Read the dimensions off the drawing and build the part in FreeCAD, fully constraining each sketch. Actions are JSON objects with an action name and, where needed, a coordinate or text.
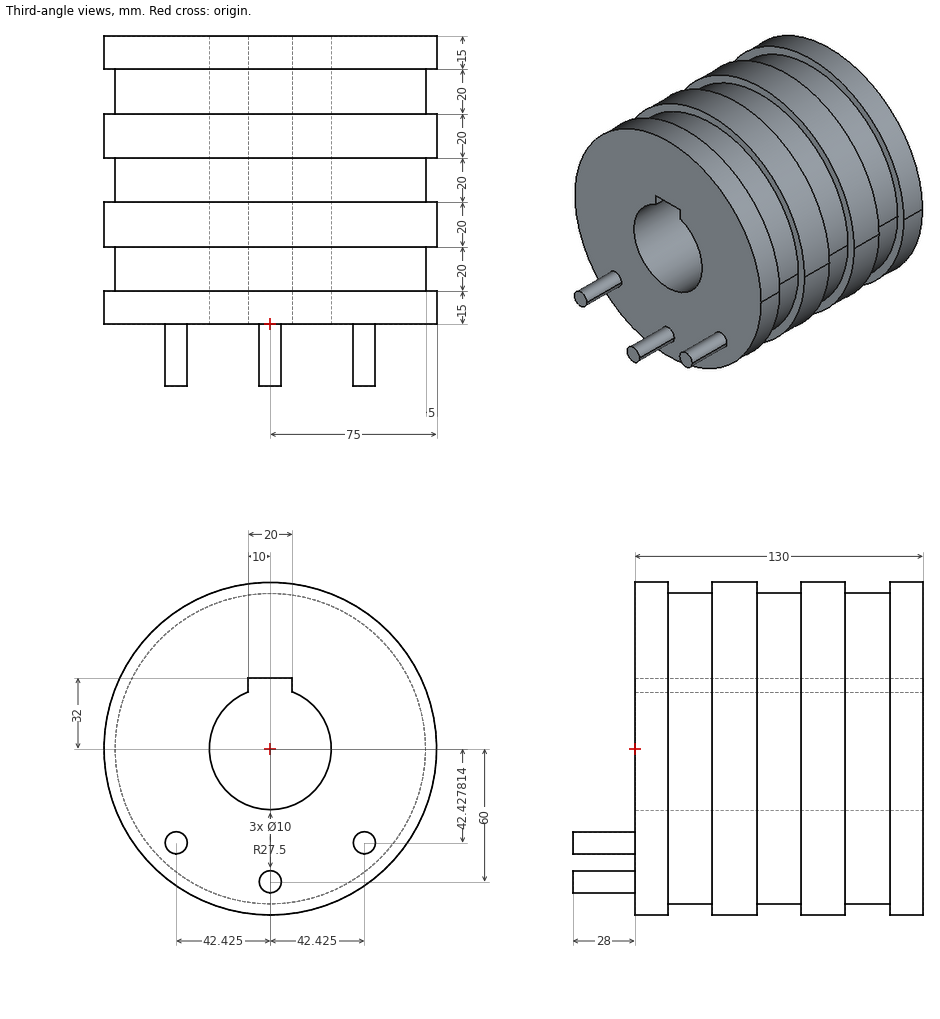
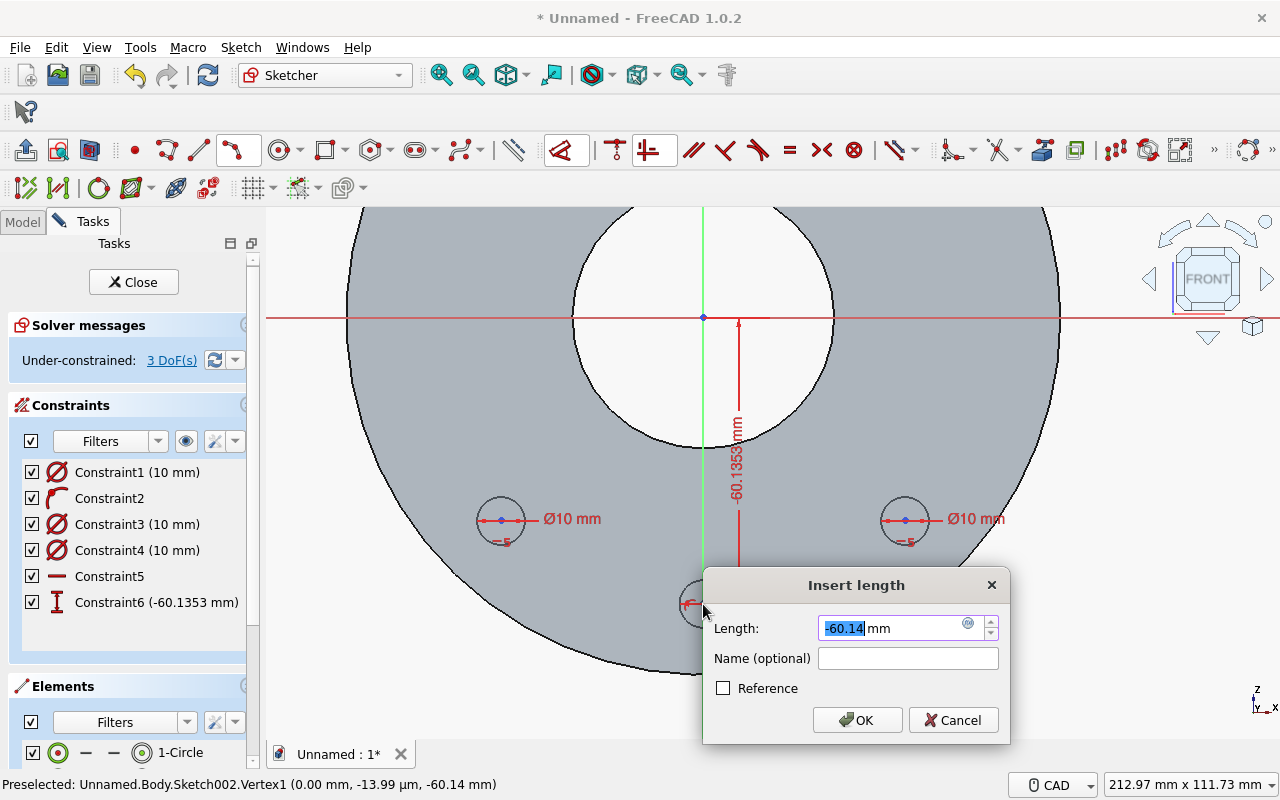
{"action": "type", "text": "-60"}
{"action": "key", "text": "Return"}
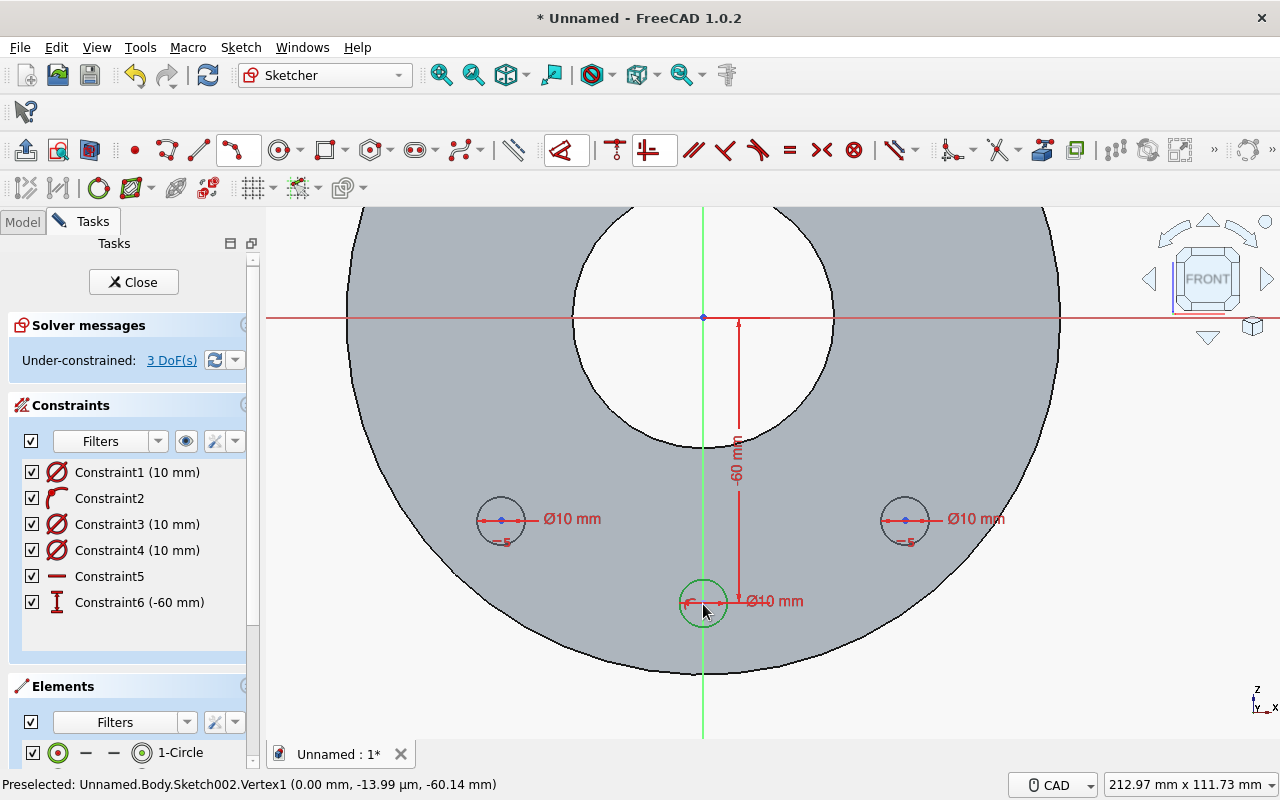
{"action": "left_click", "coordinate": [905, 521]}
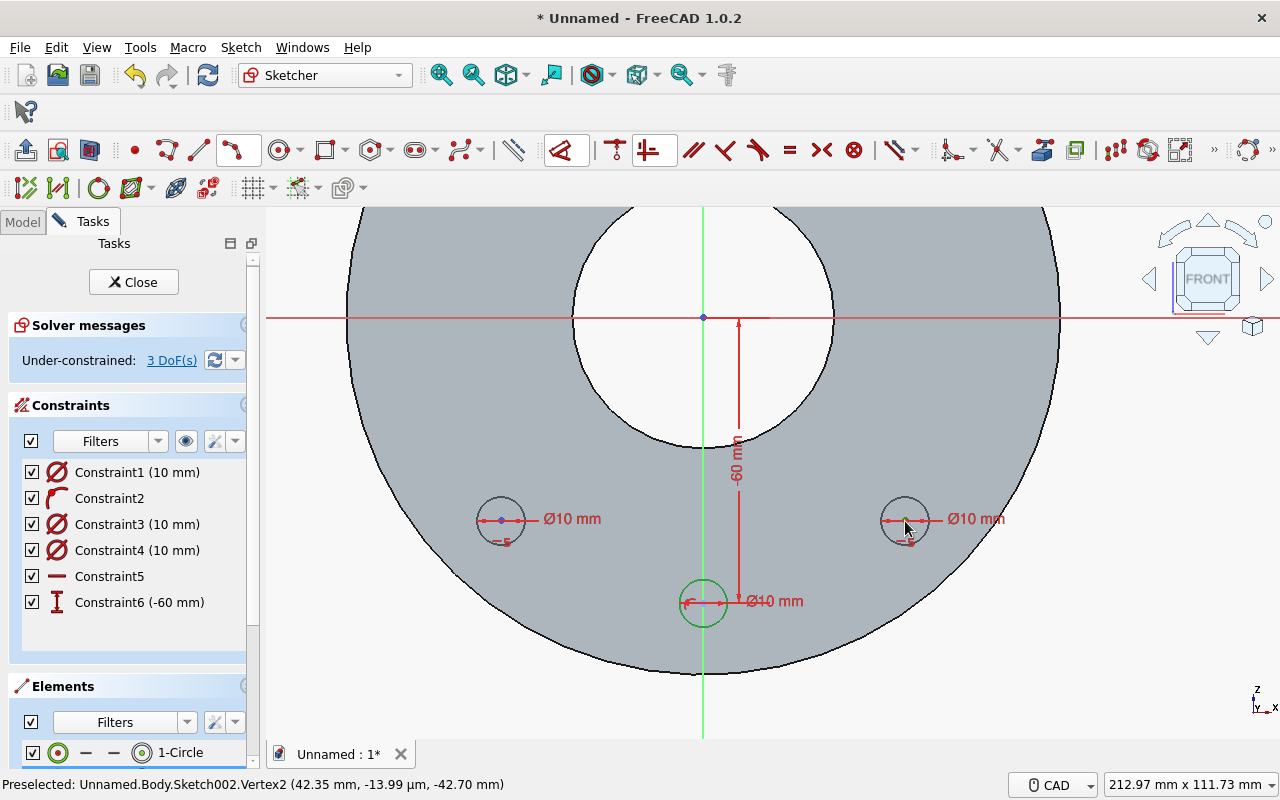
{"action": "key", "text": "l"}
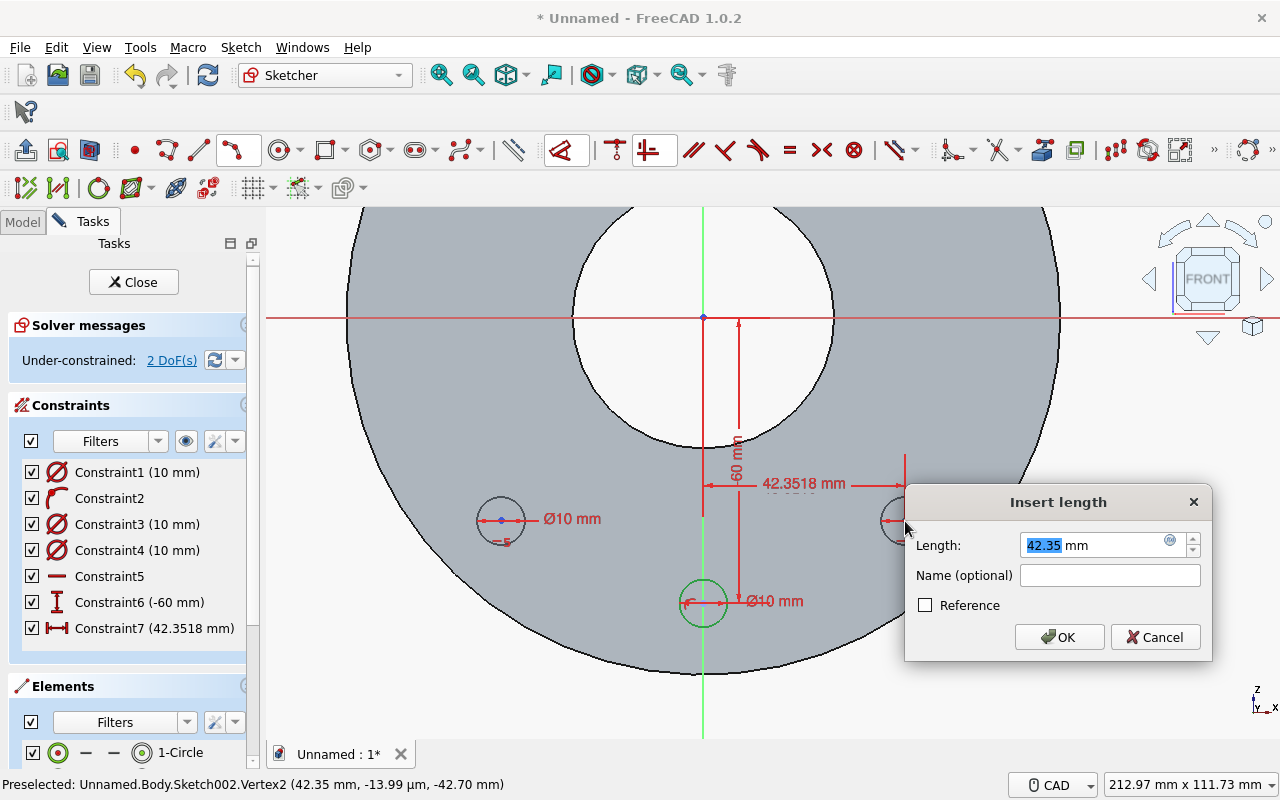
{"action": "type", "text": "42.425"}
{"action": "key", "text": "Return"}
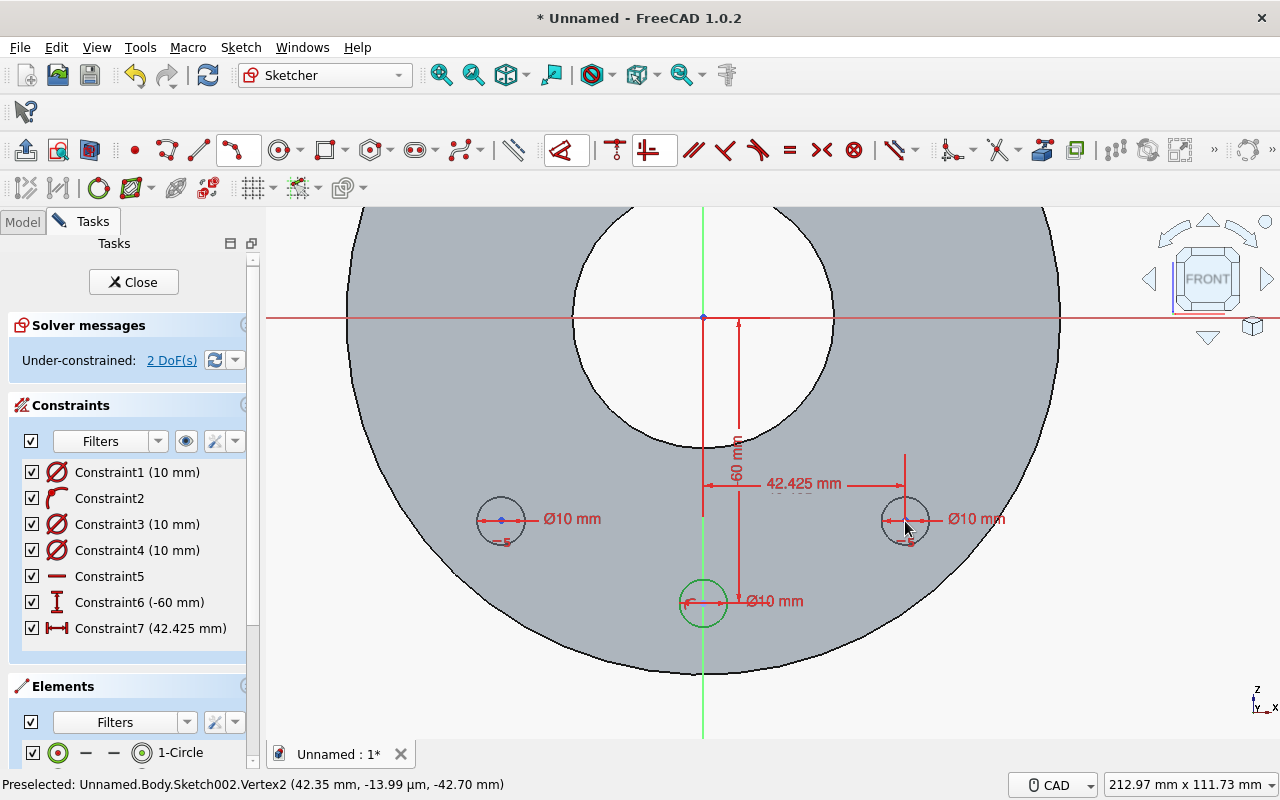
{"action": "left_click", "coordinate": [501, 521]}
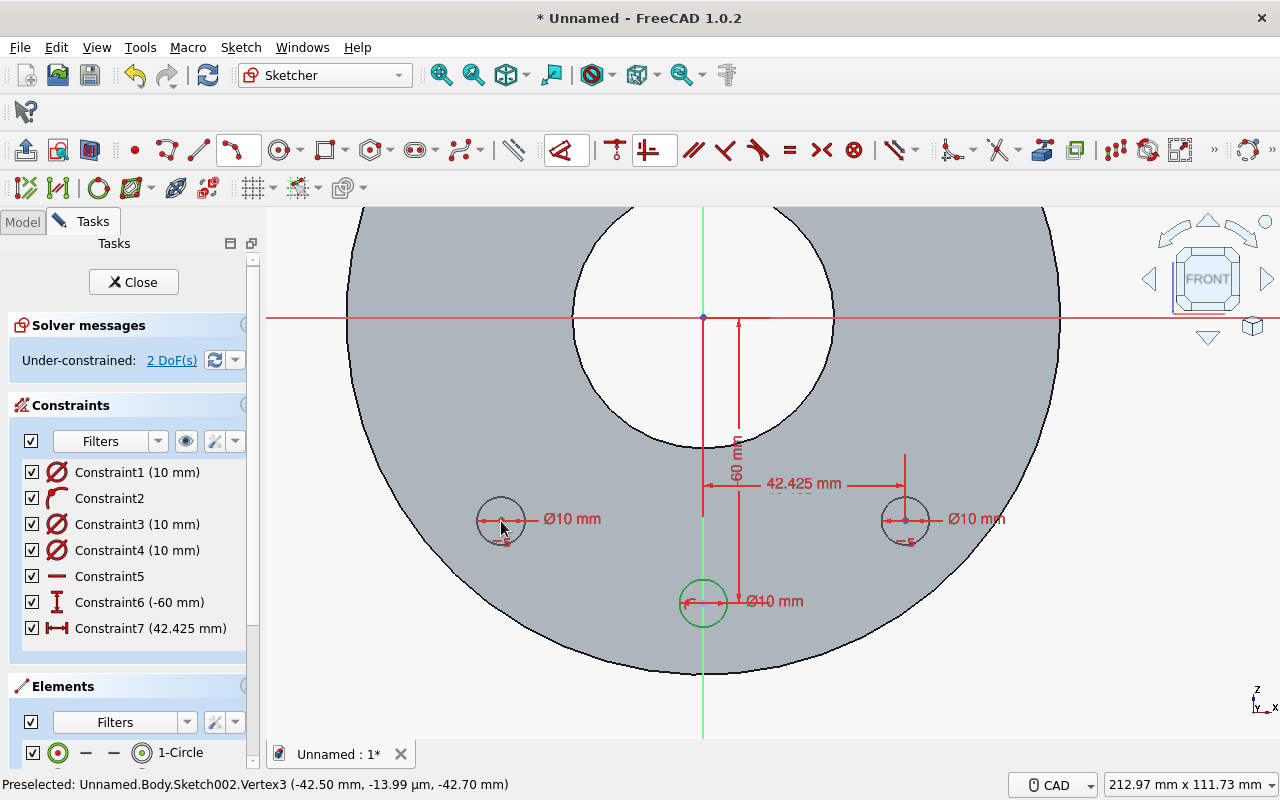
{"action": "key", "text": "l"}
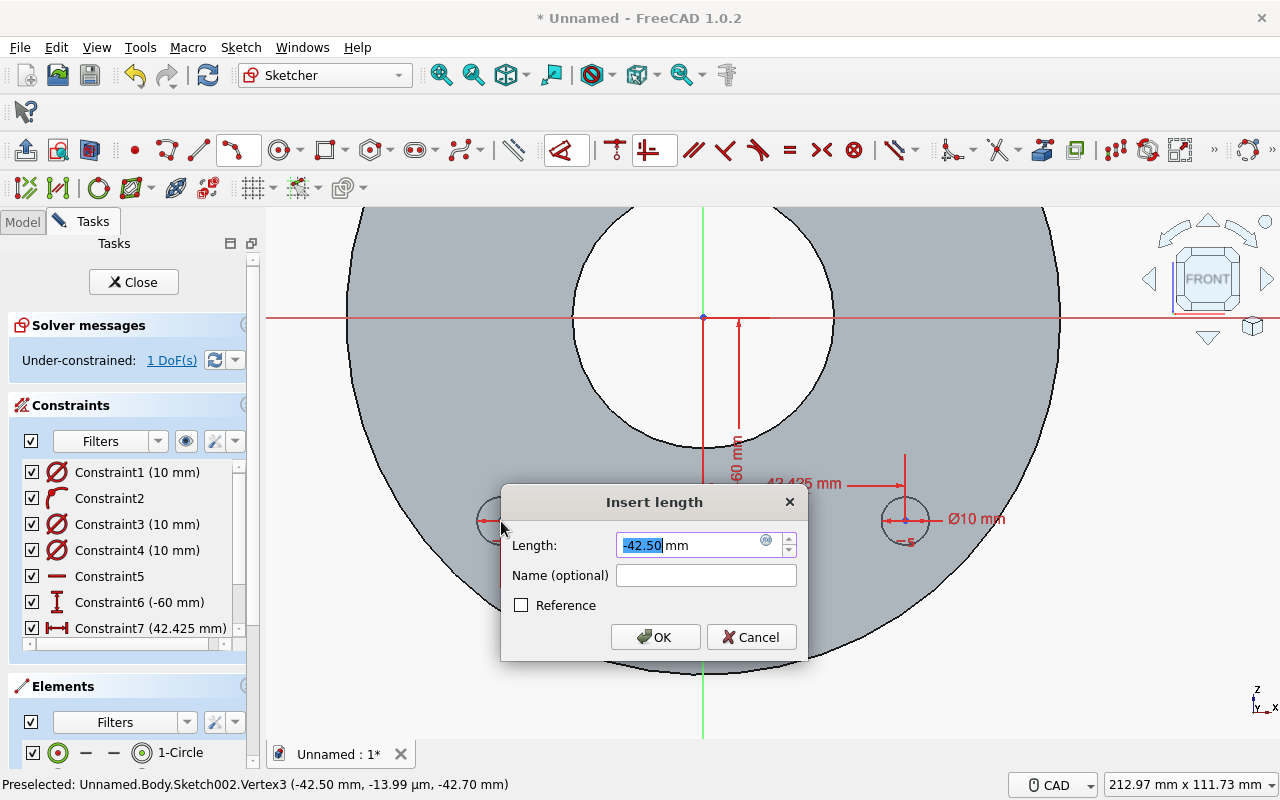
{"action": "type", "text": "-42.425"}
{"action": "key", "text": "Return"}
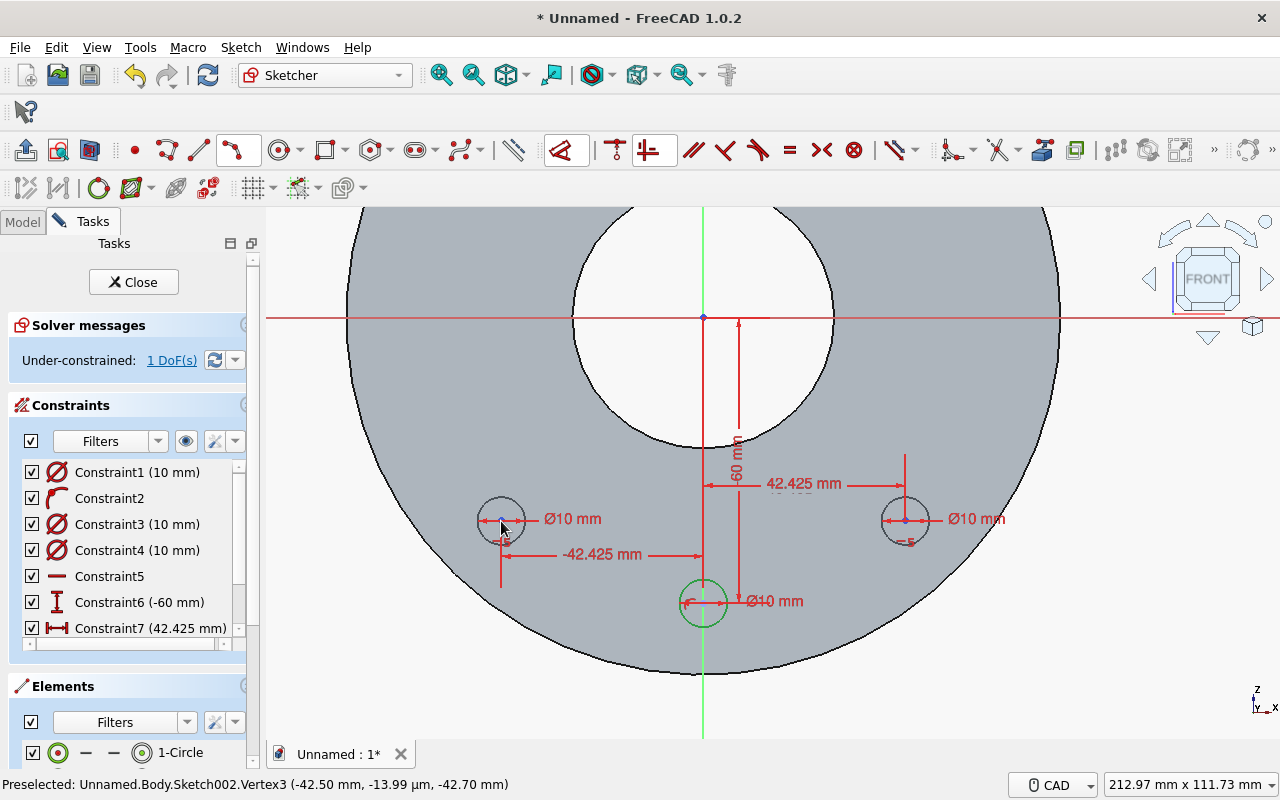
{"action": "left_click", "coordinate": [905, 521]}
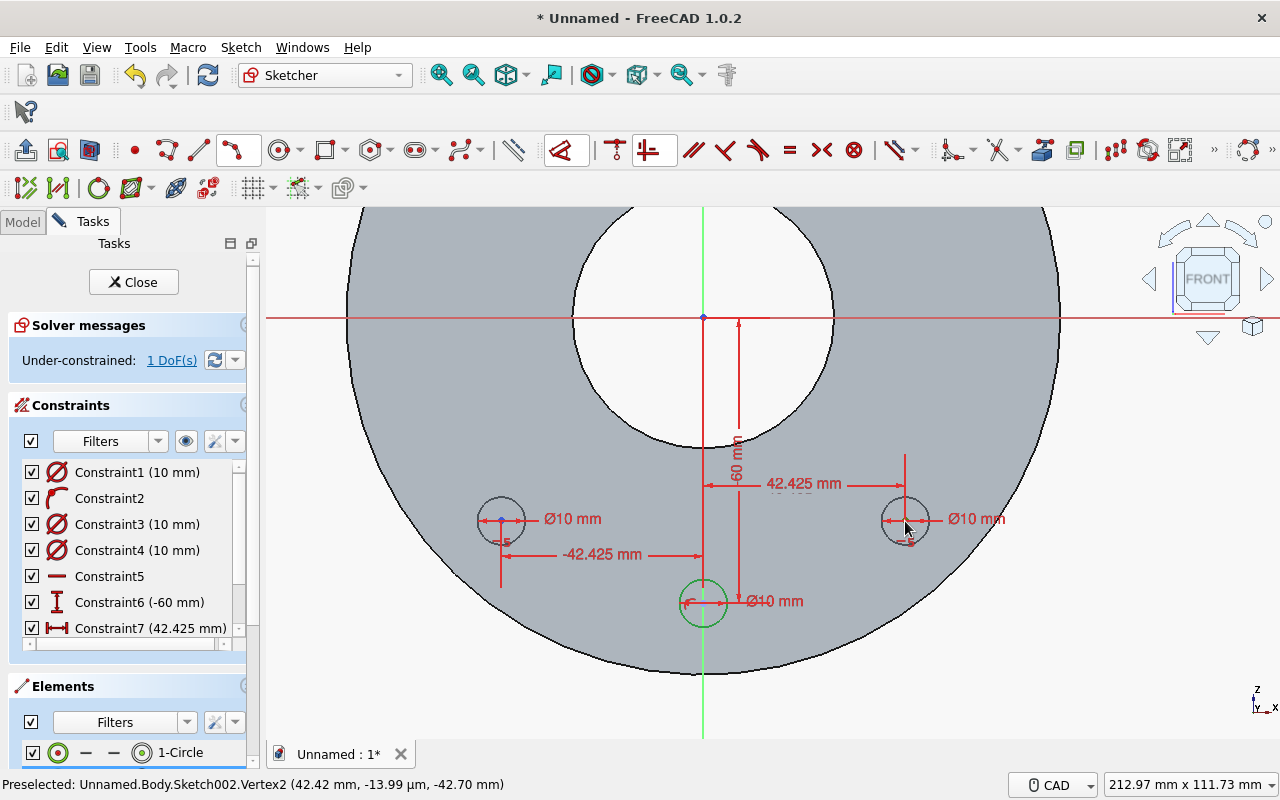
{"action": "key", "text": "i"}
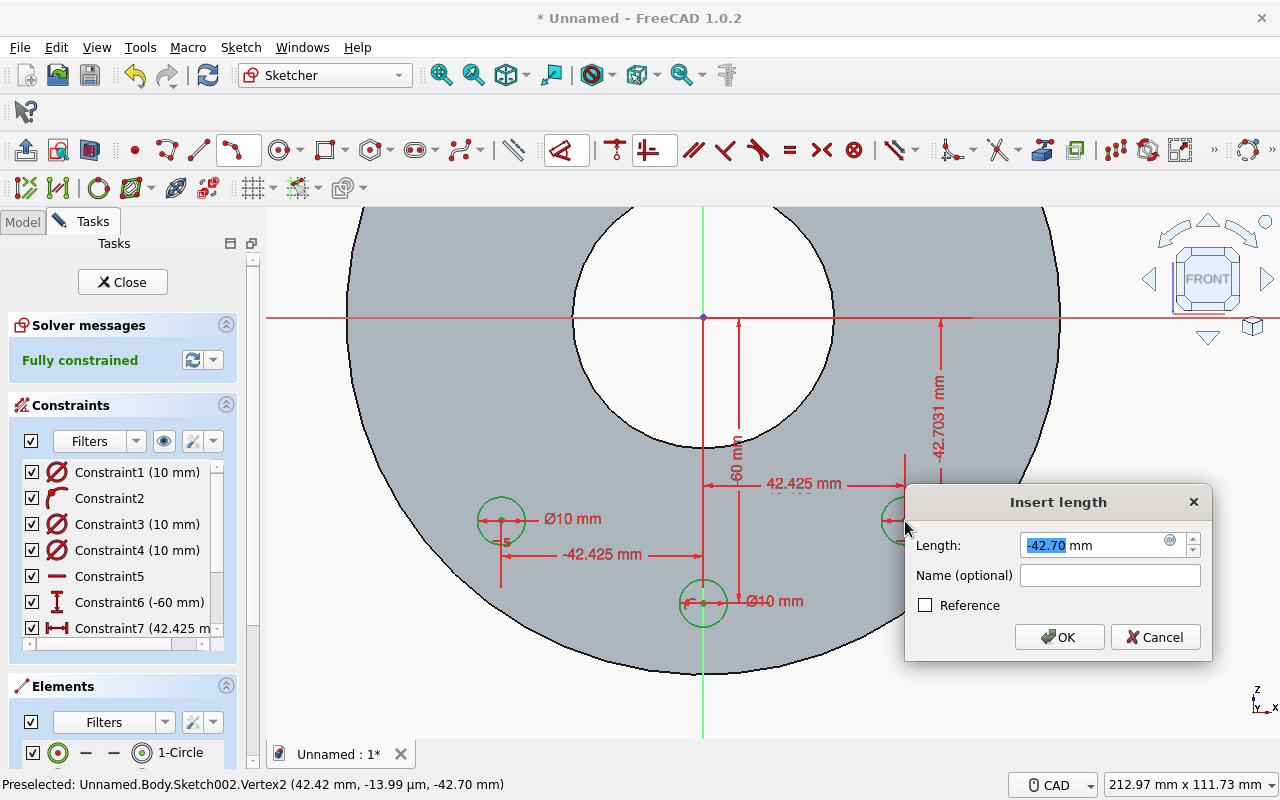
{"action": "type", "text": "-42.427814"}
{"action": "key", "text": "Return"}